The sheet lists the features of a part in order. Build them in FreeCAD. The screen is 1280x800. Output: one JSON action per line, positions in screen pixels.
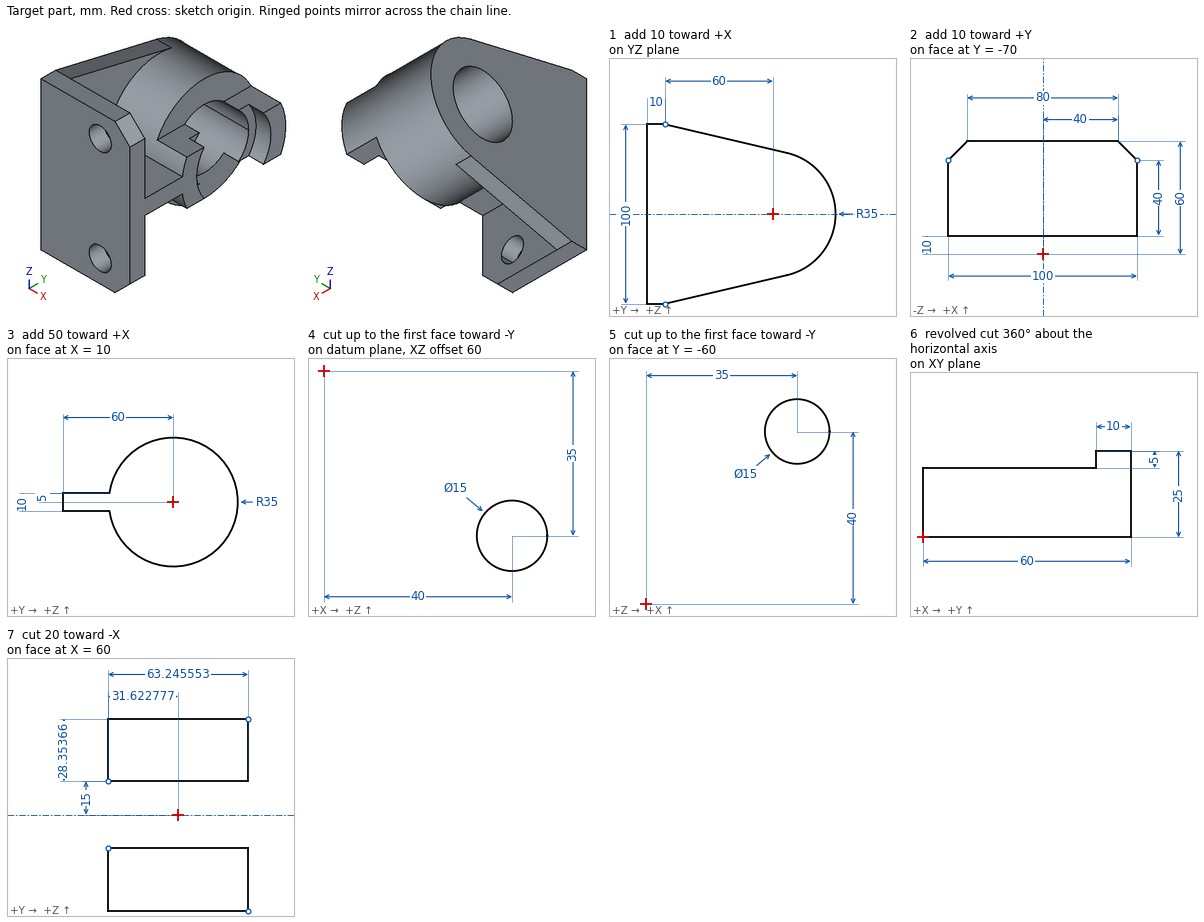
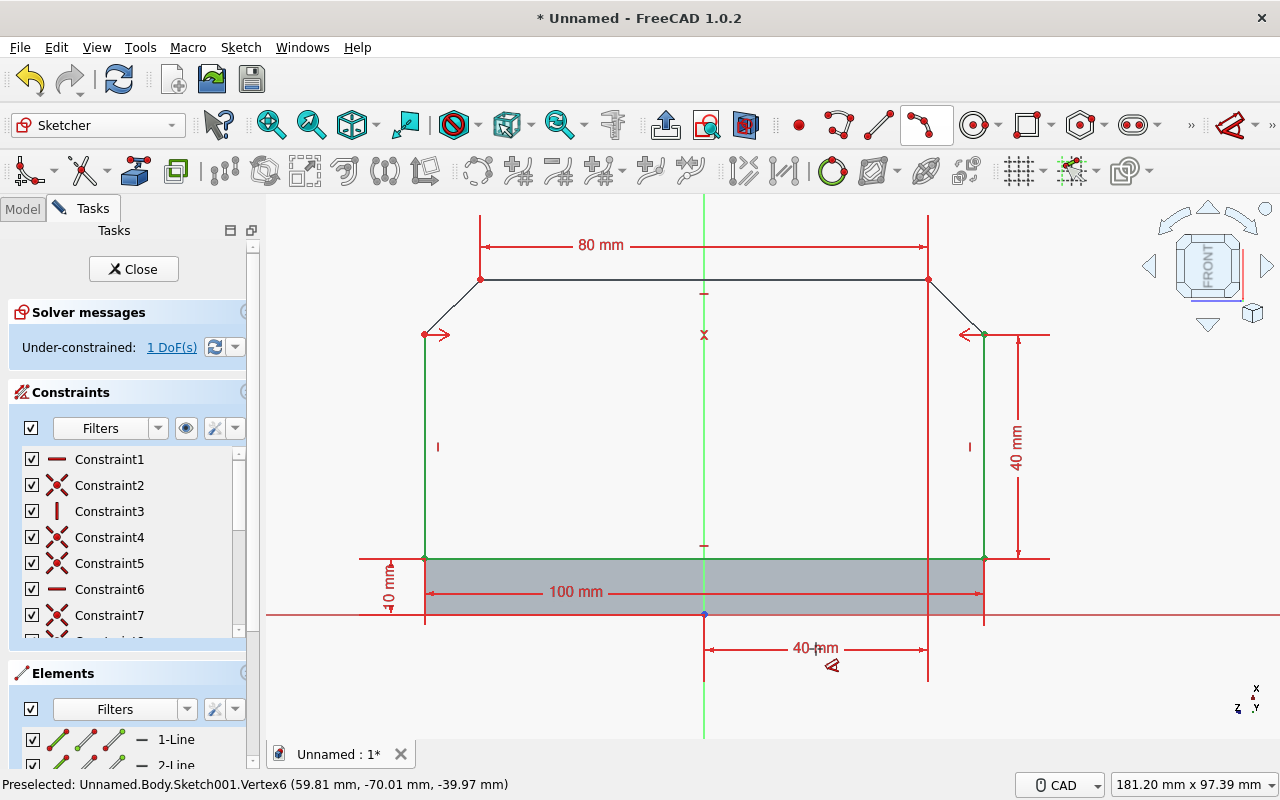
{"action": "left_click", "coordinate": [928, 280]}
{"action": "left_click", "coordinate": [962, 370]}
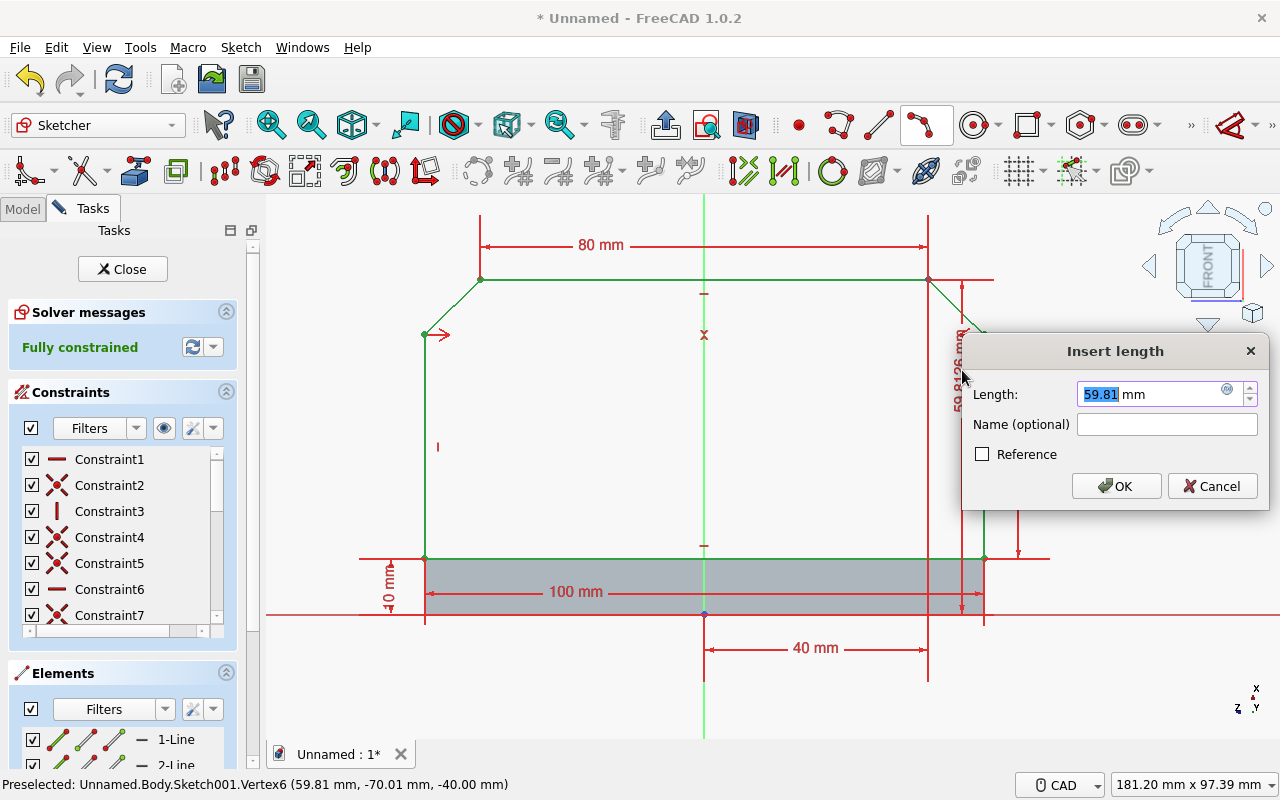
{"action": "type", "text": "60"}
{"action": "key", "text": "Return"}
{"action": "key", "text": "Escape"}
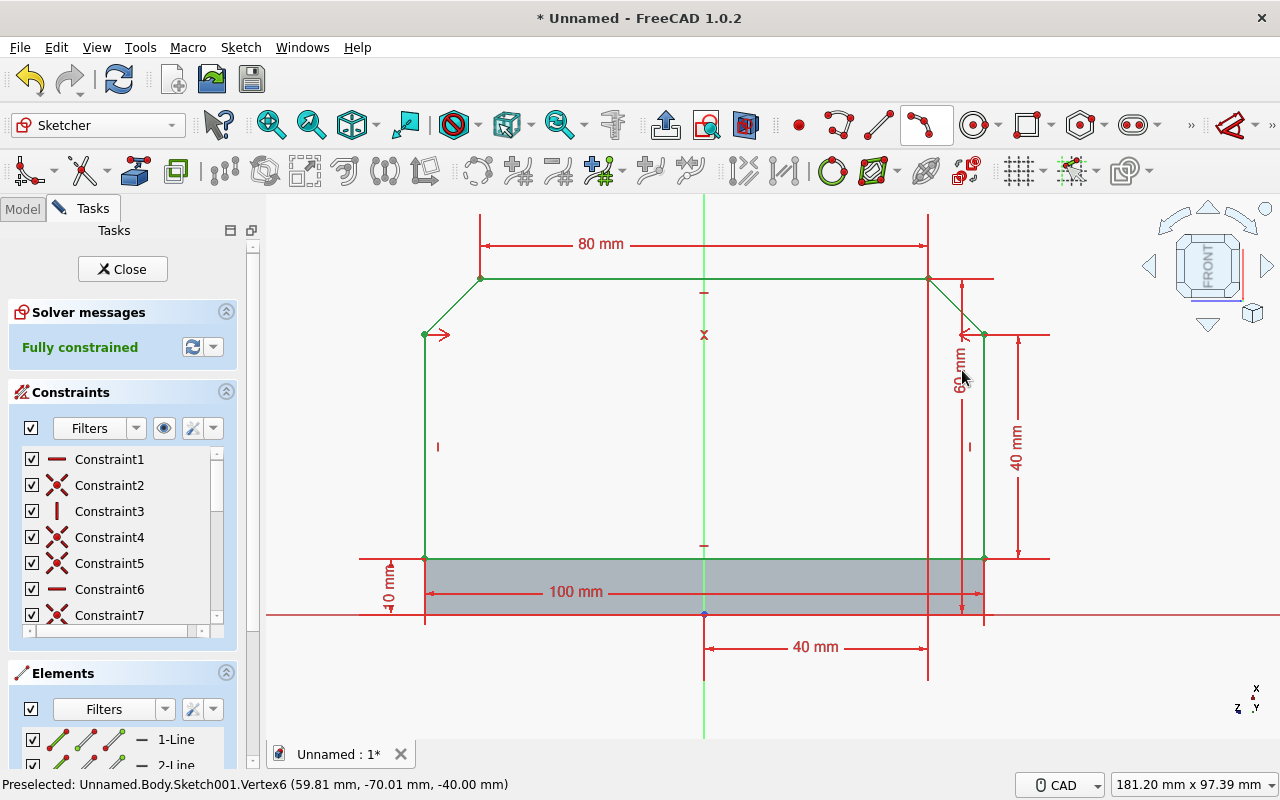
{"action": "left_click", "coordinate": [123, 269]}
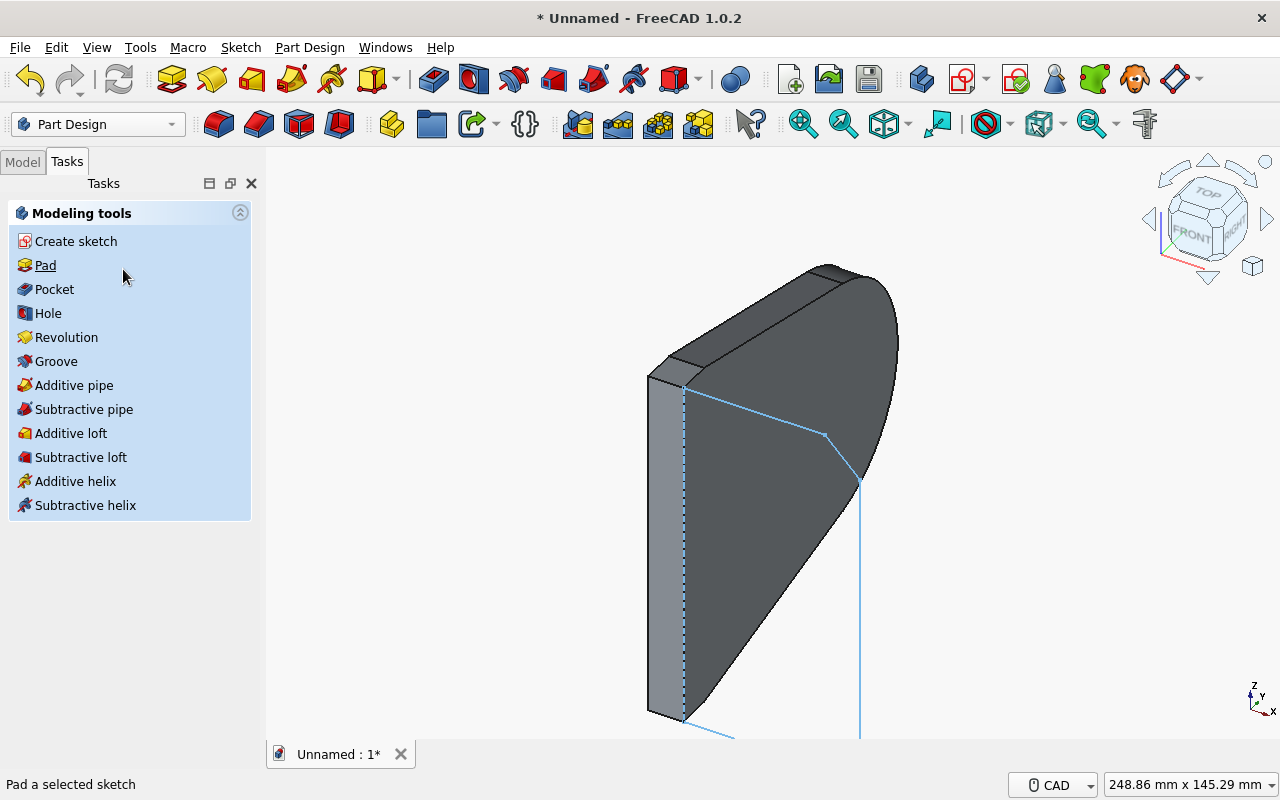
{"action": "left_click", "coordinate": [172, 80]}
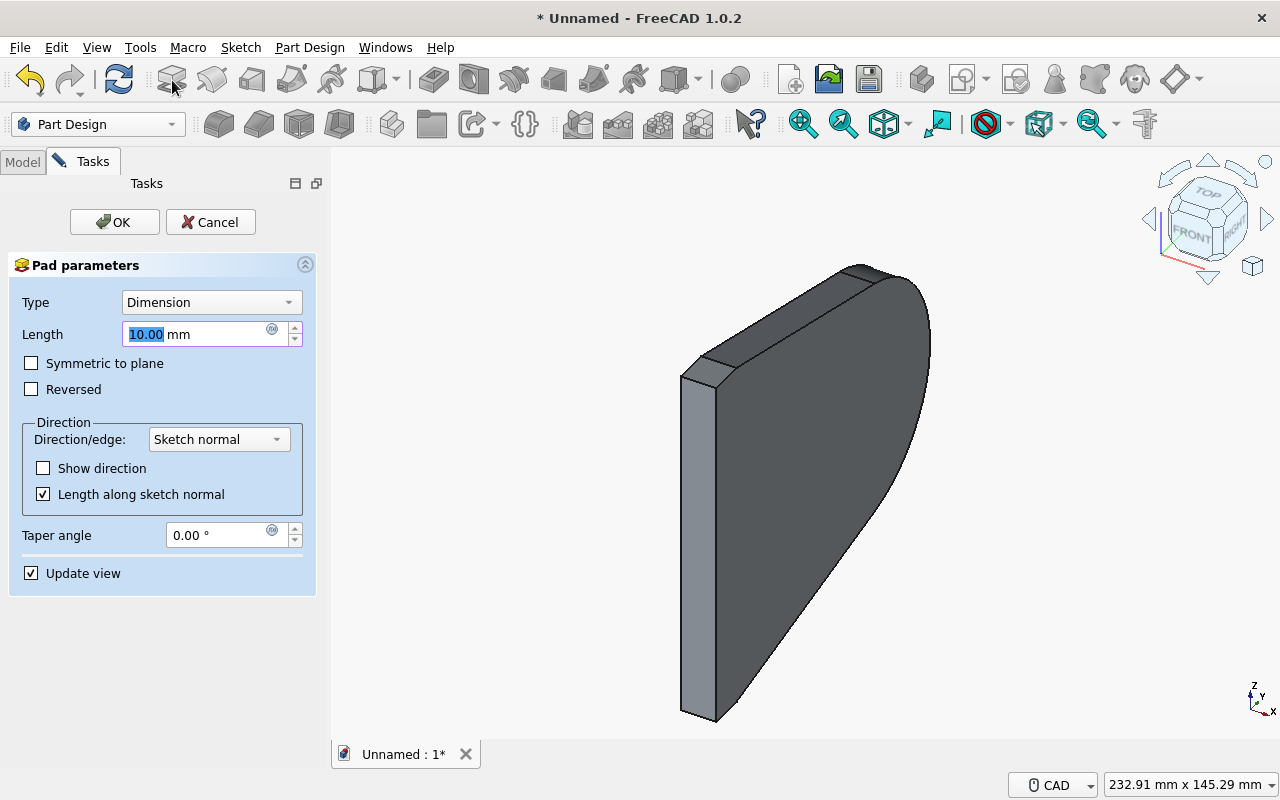
{"action": "type", "text": "10"}
{"action": "key", "text": "Tab"}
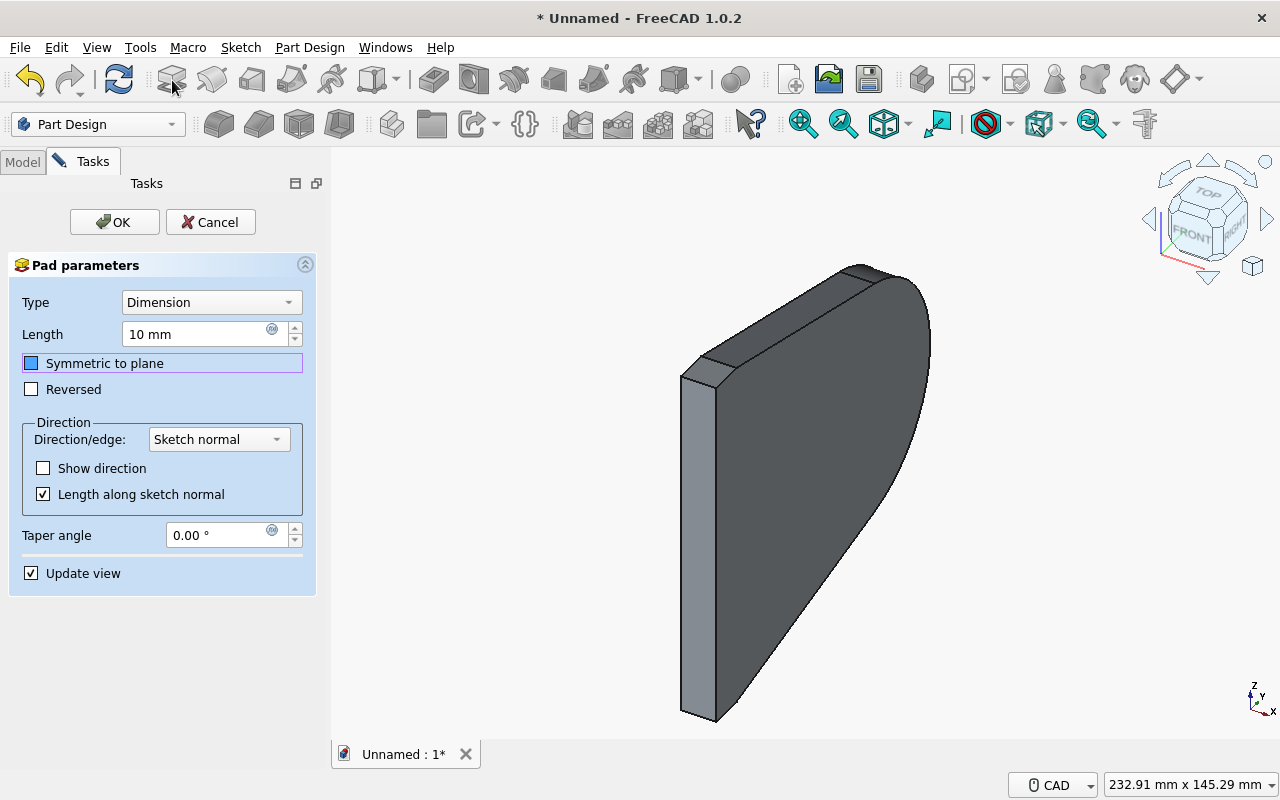
{"action": "left_click", "coordinate": [30, 389]}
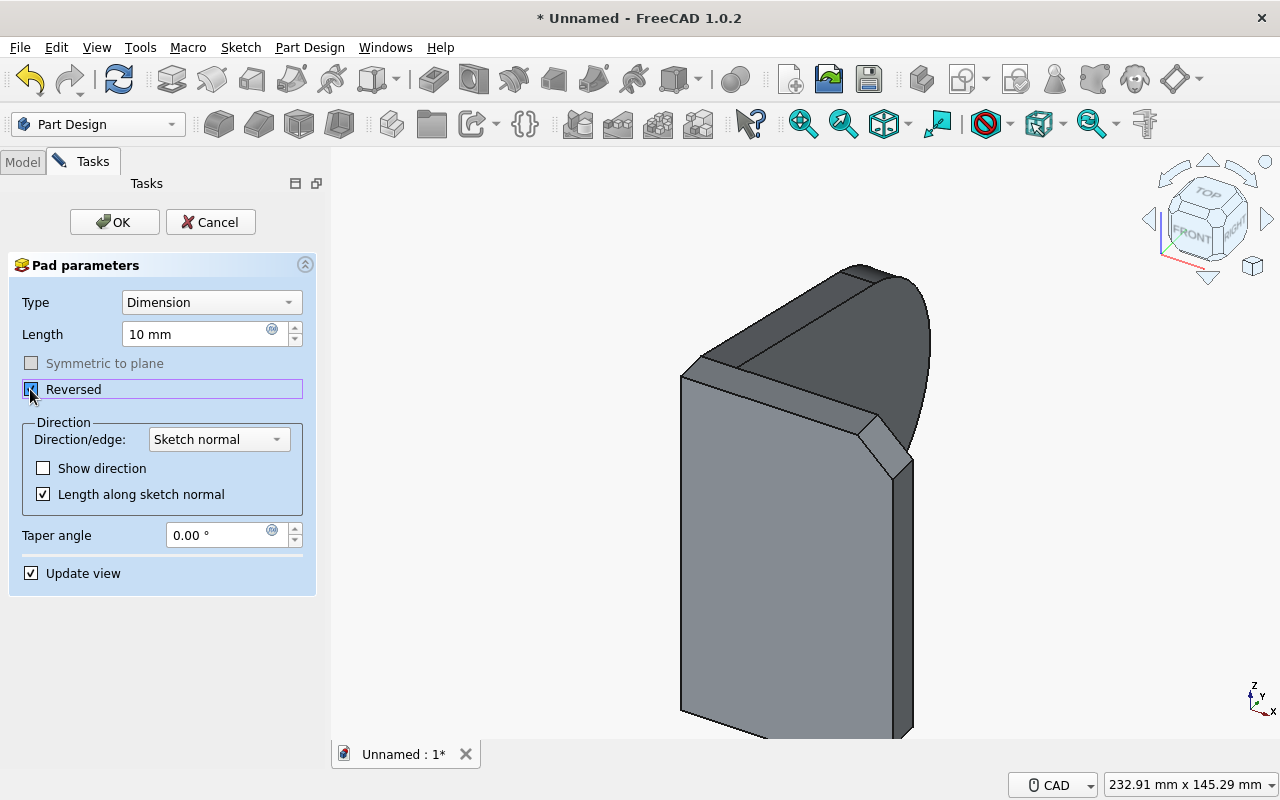
{"action": "left_click", "coordinate": [115, 222]}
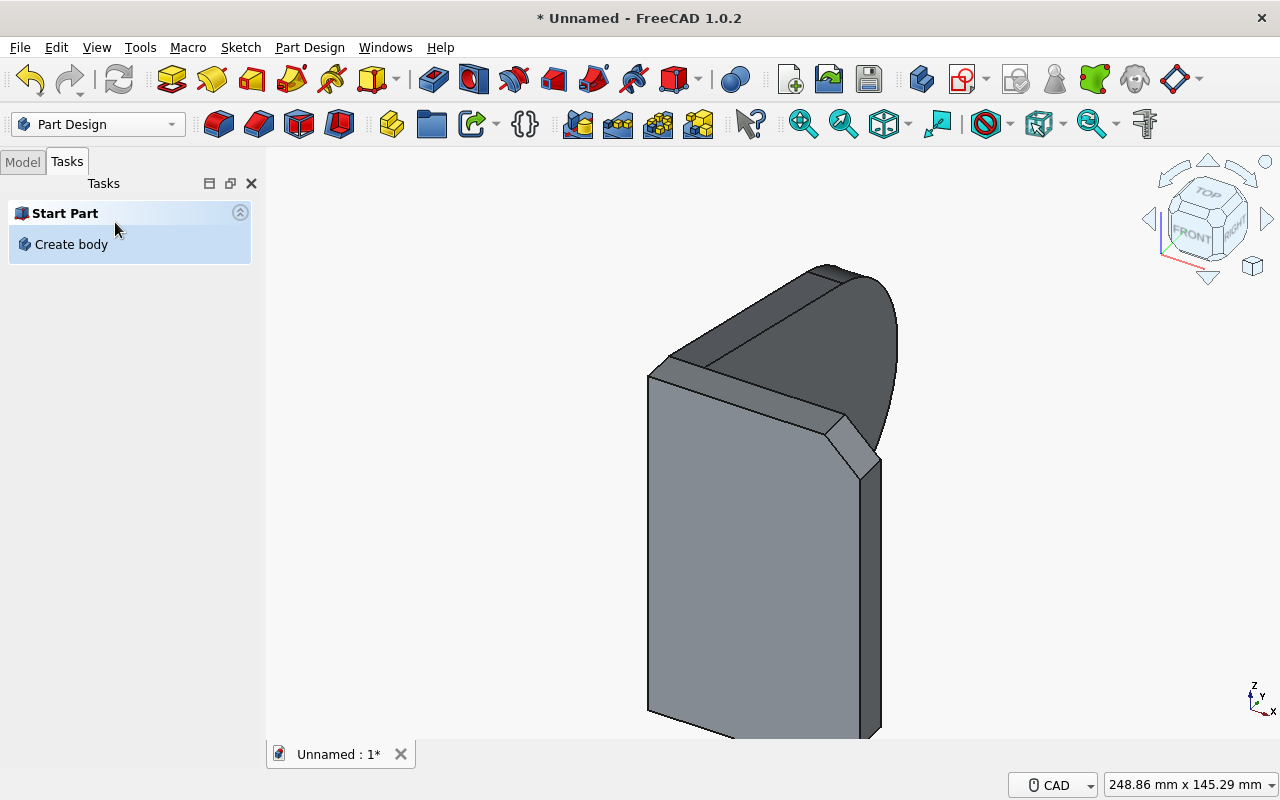
{"action": "left_click", "coordinate": [804, 124]}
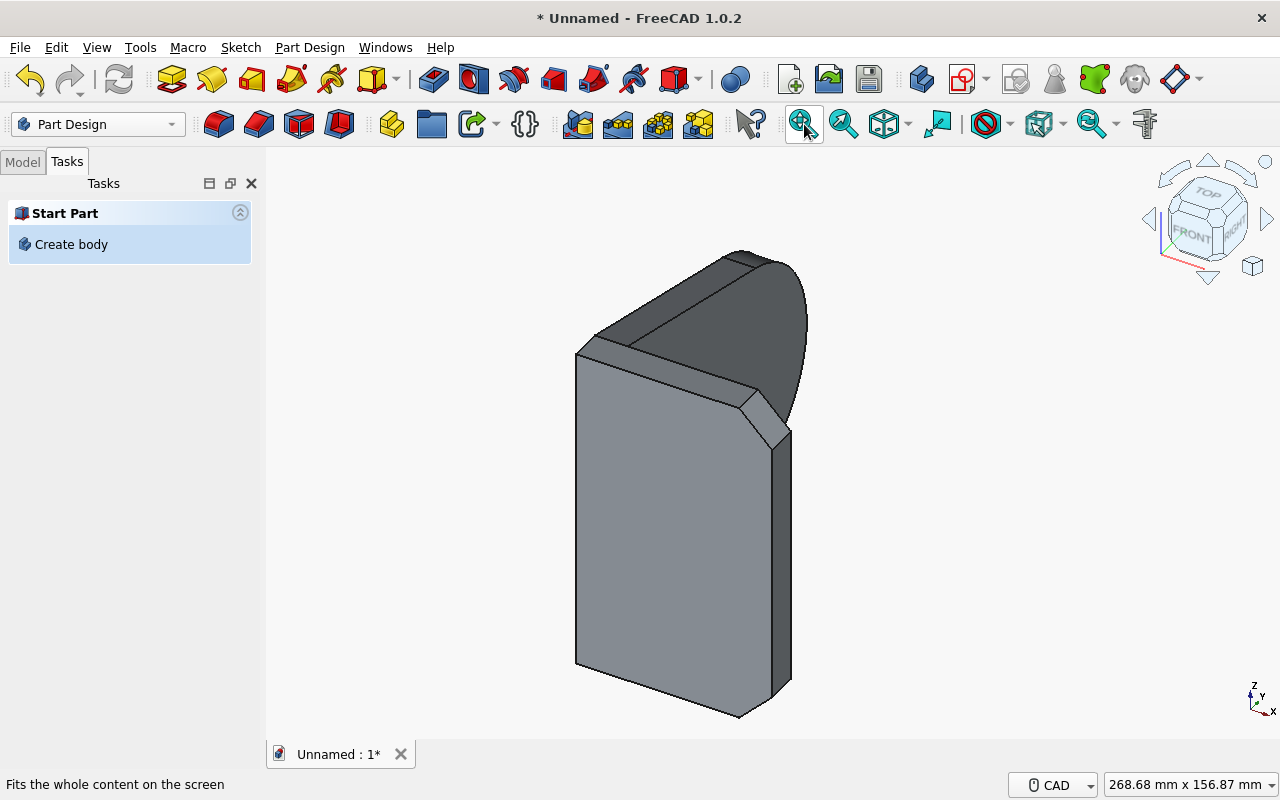
{"action": "key", "text": "0"}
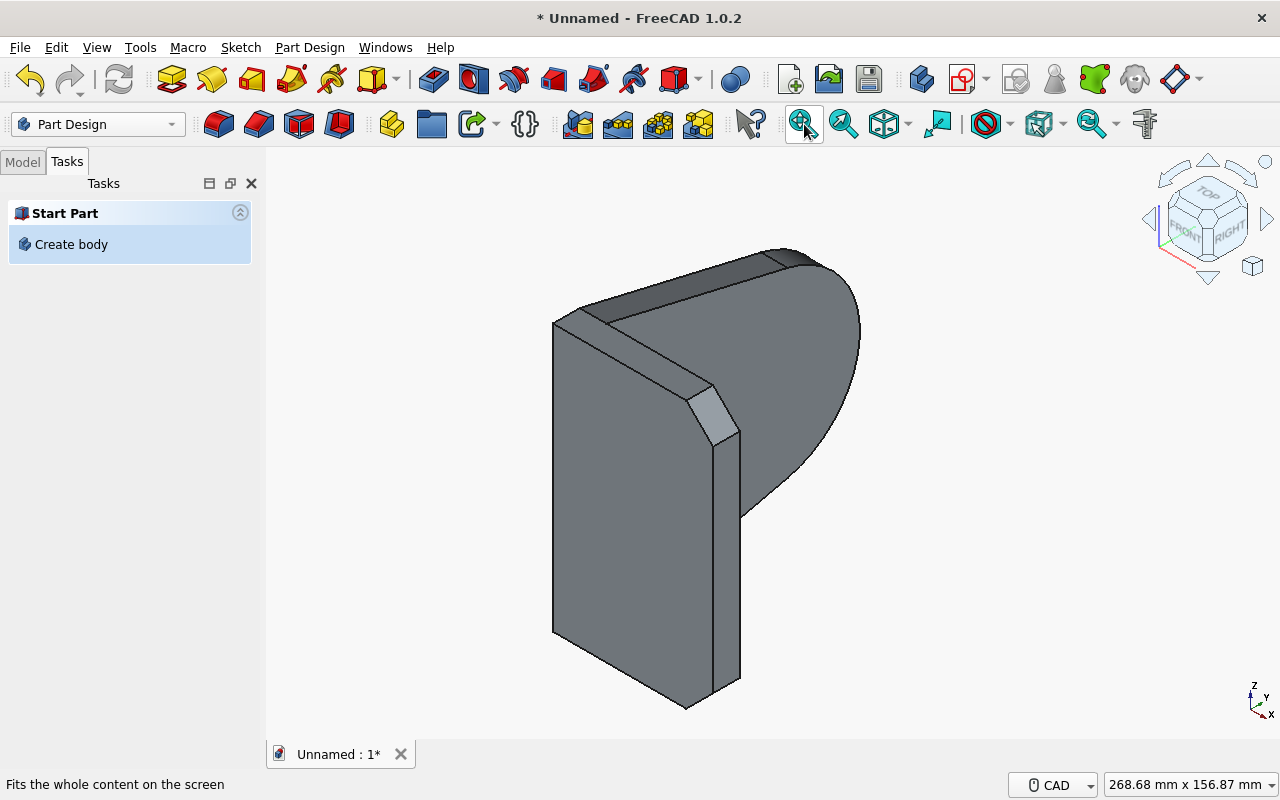
{"action": "left_click", "coordinate": [769, 383]}